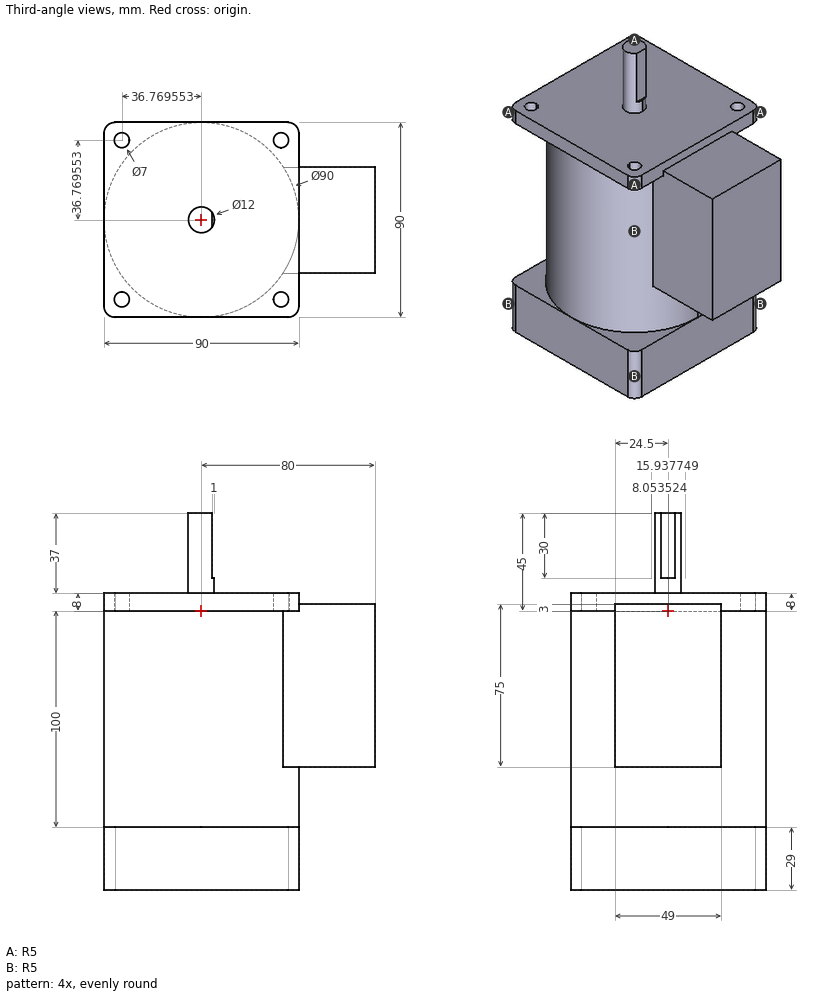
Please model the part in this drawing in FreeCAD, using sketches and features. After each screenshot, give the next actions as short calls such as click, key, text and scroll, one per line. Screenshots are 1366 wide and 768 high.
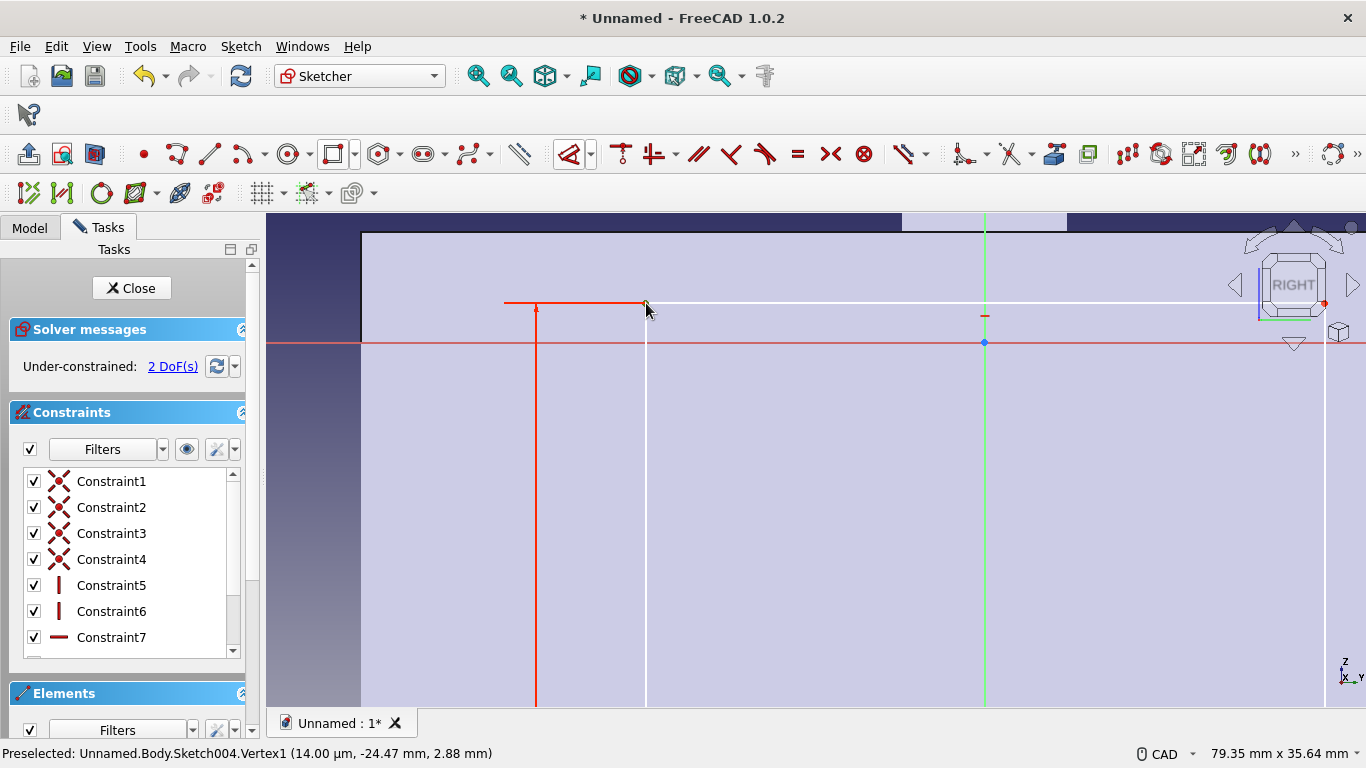
key(i)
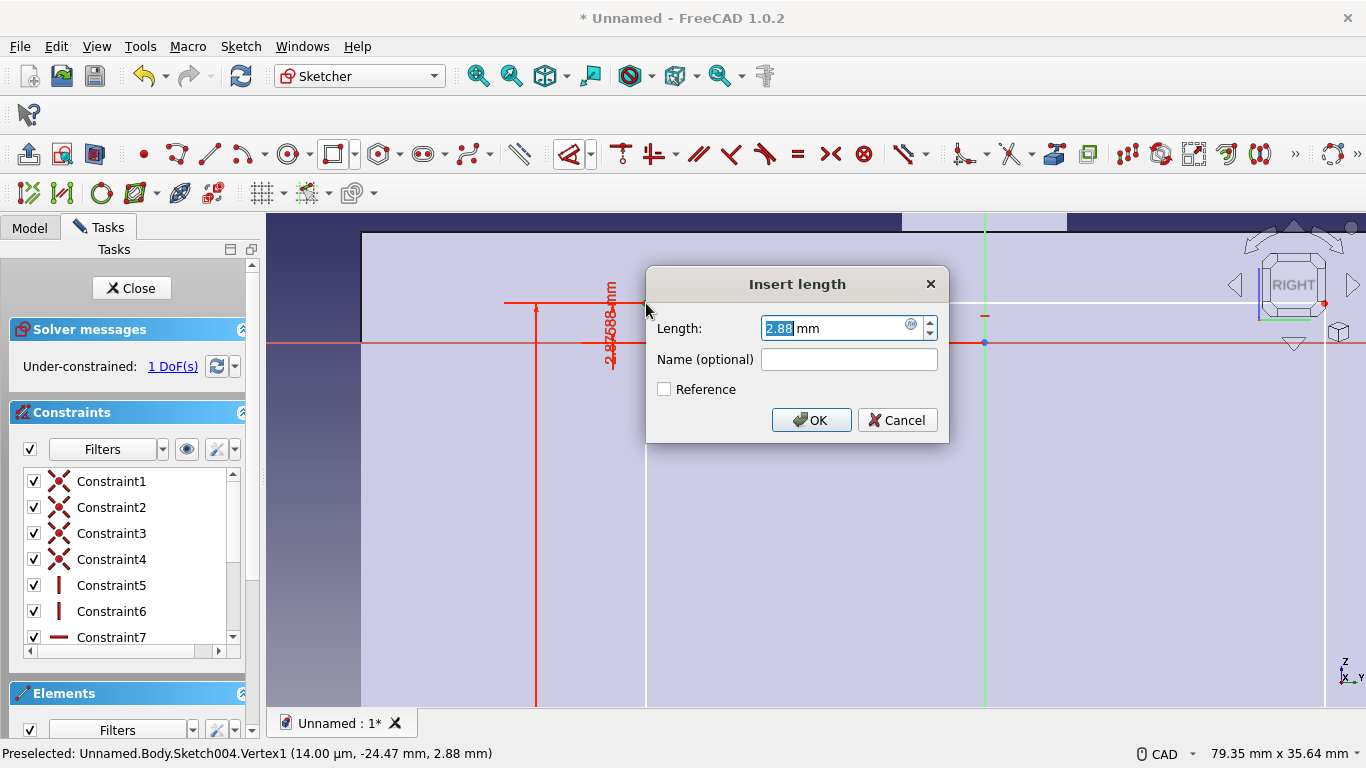
text(3)
key(Return)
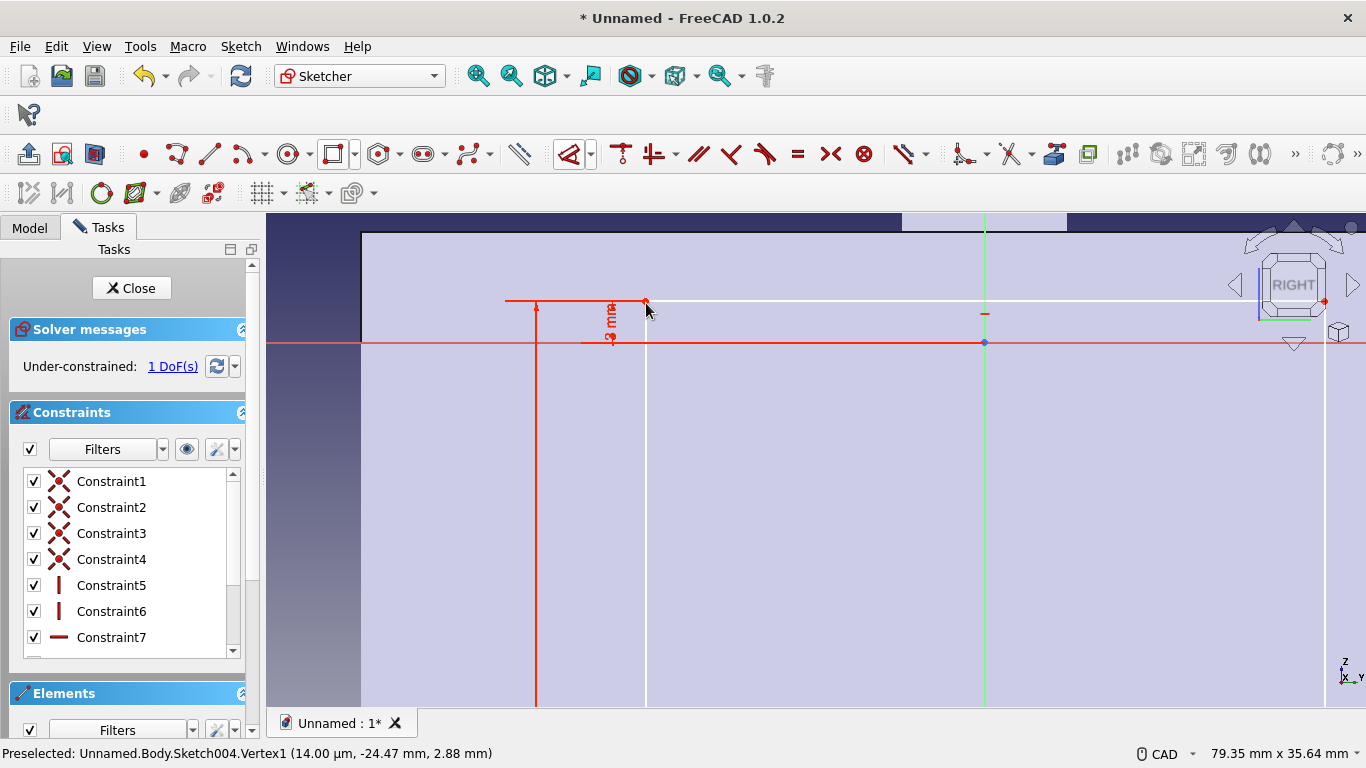
click(646, 301)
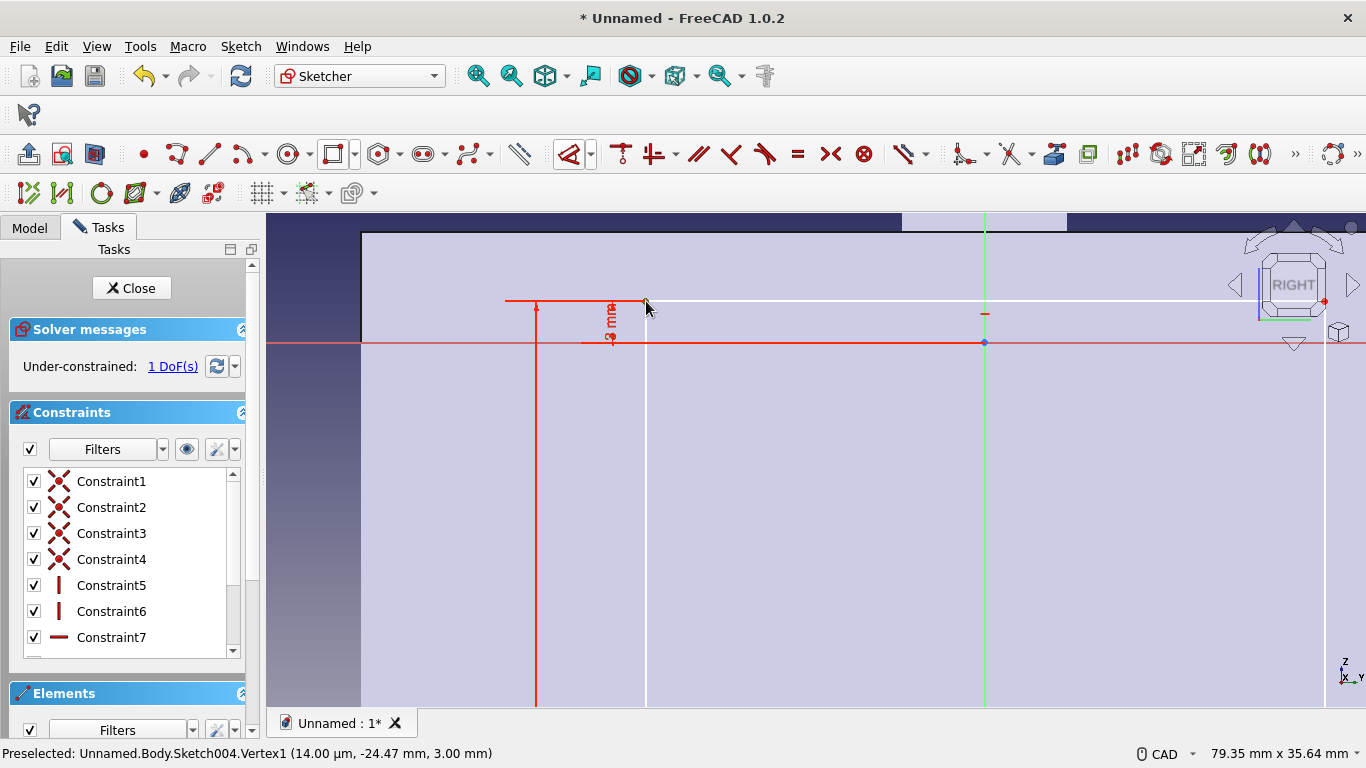
key(l)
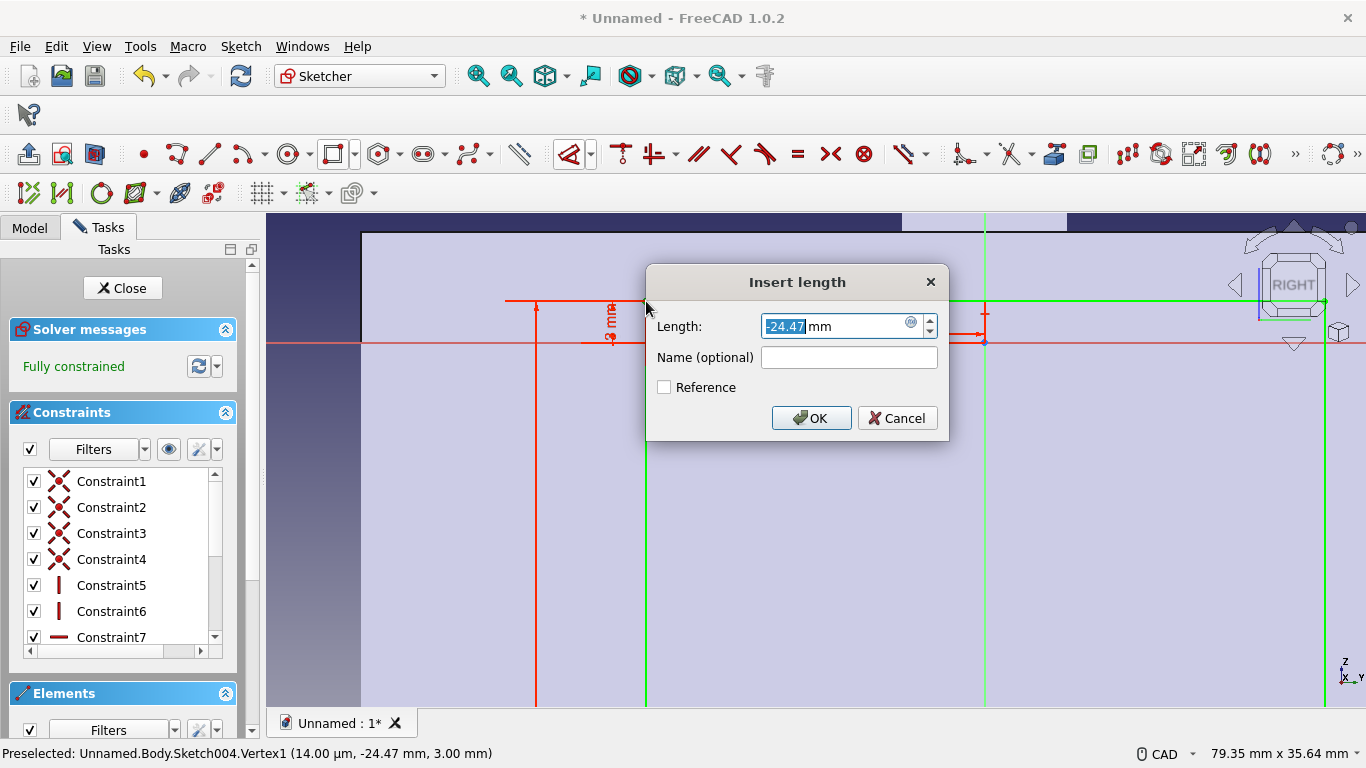
text(-24.5)
key(Return)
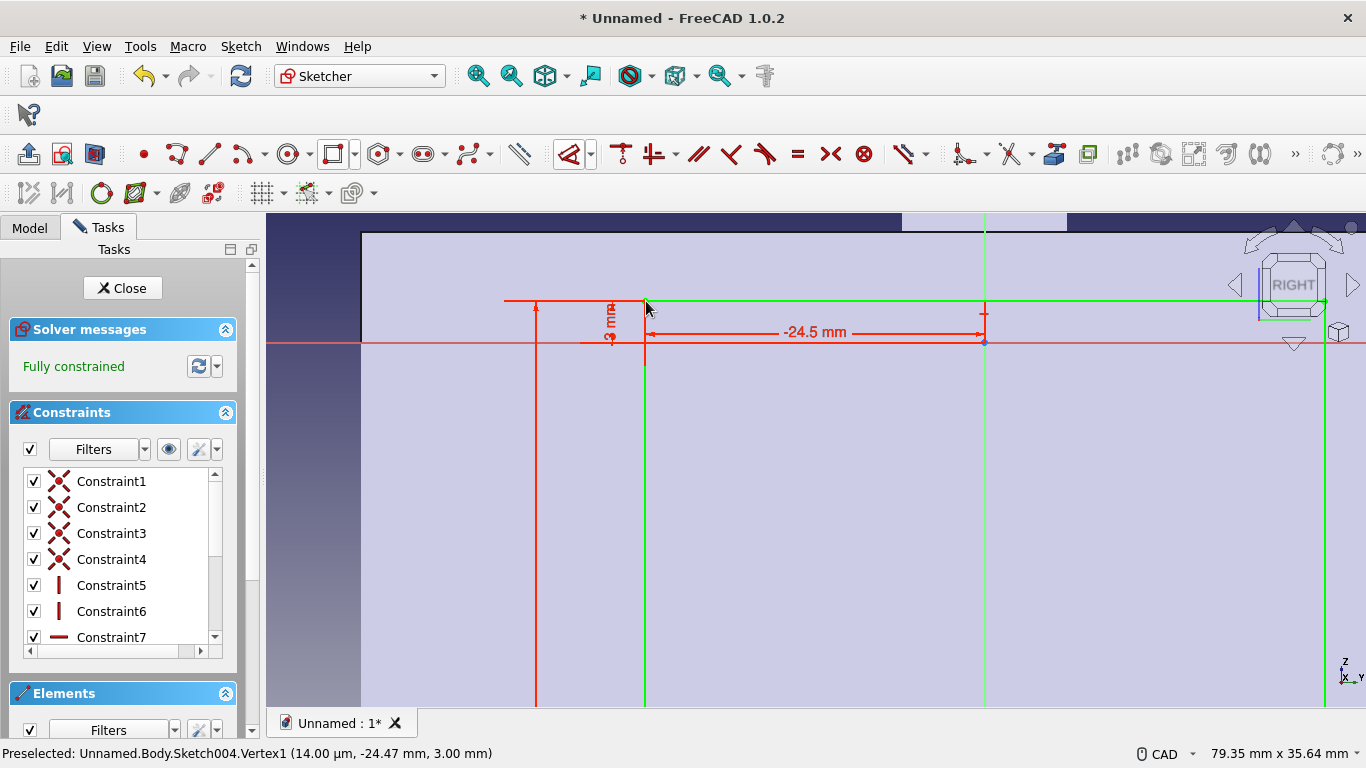
click(123, 288)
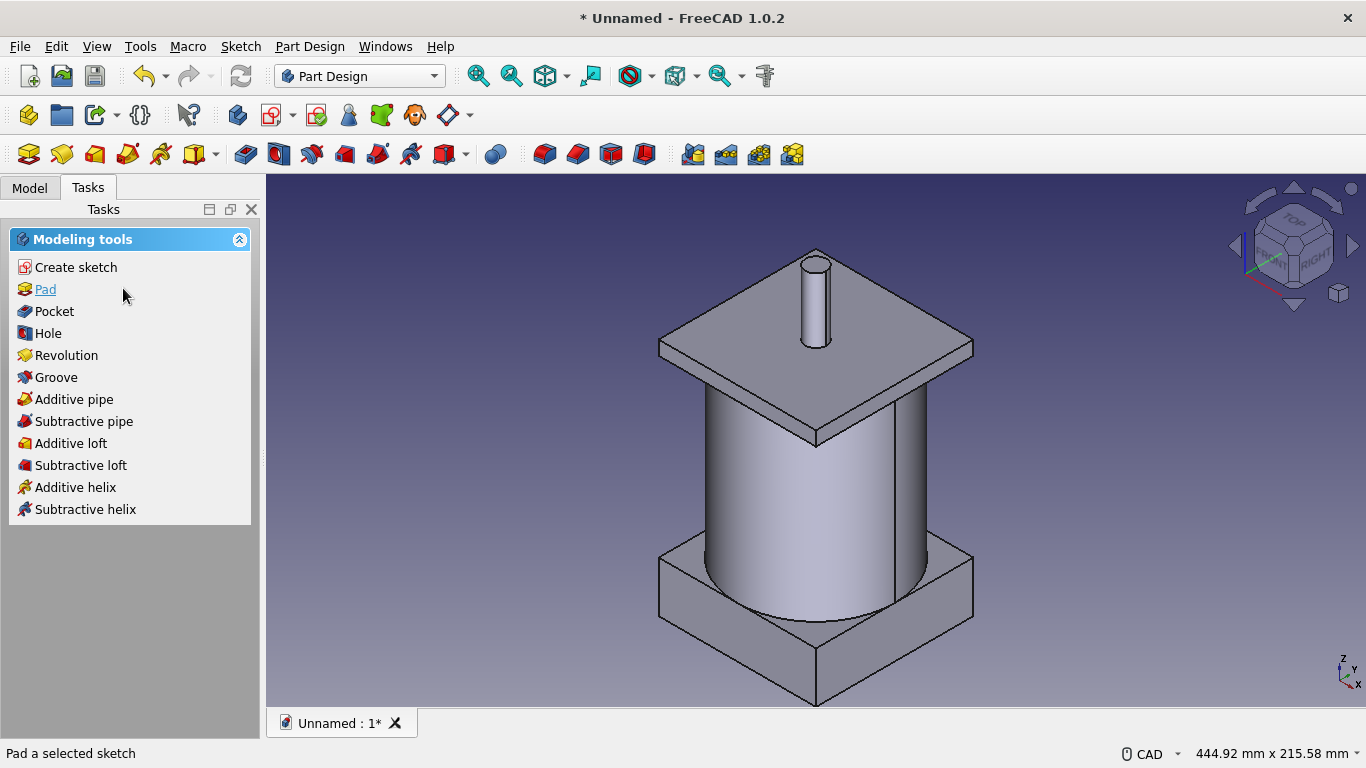
click(29, 154)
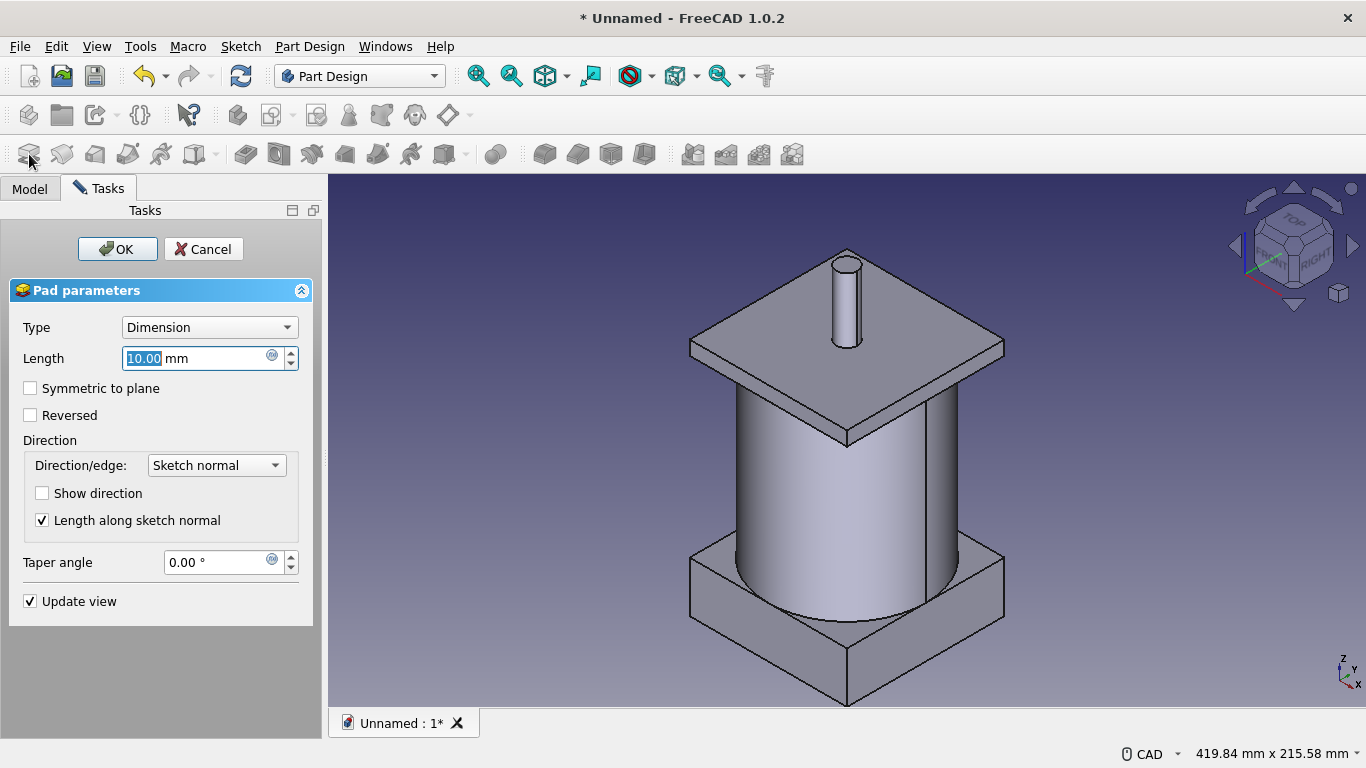
text(80)
key(Tab)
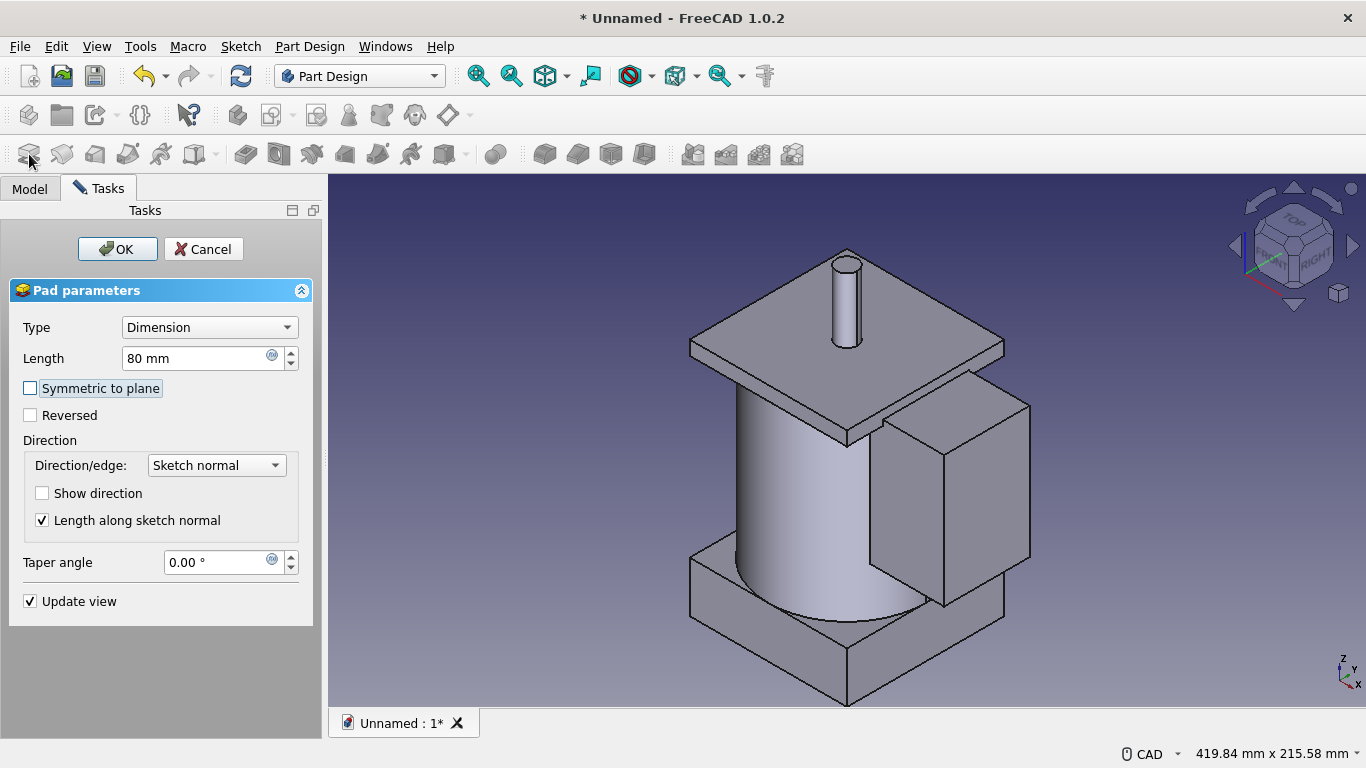
click(118, 249)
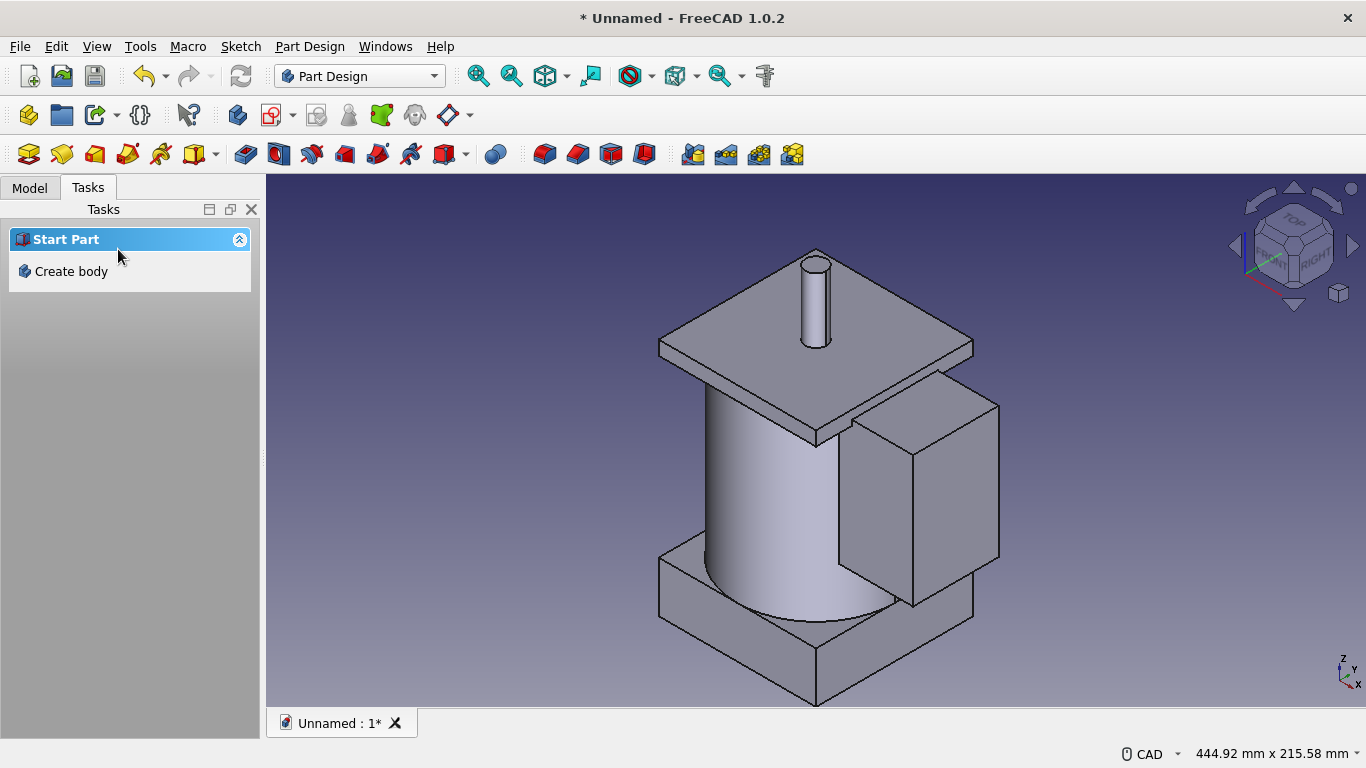
click(479, 76)